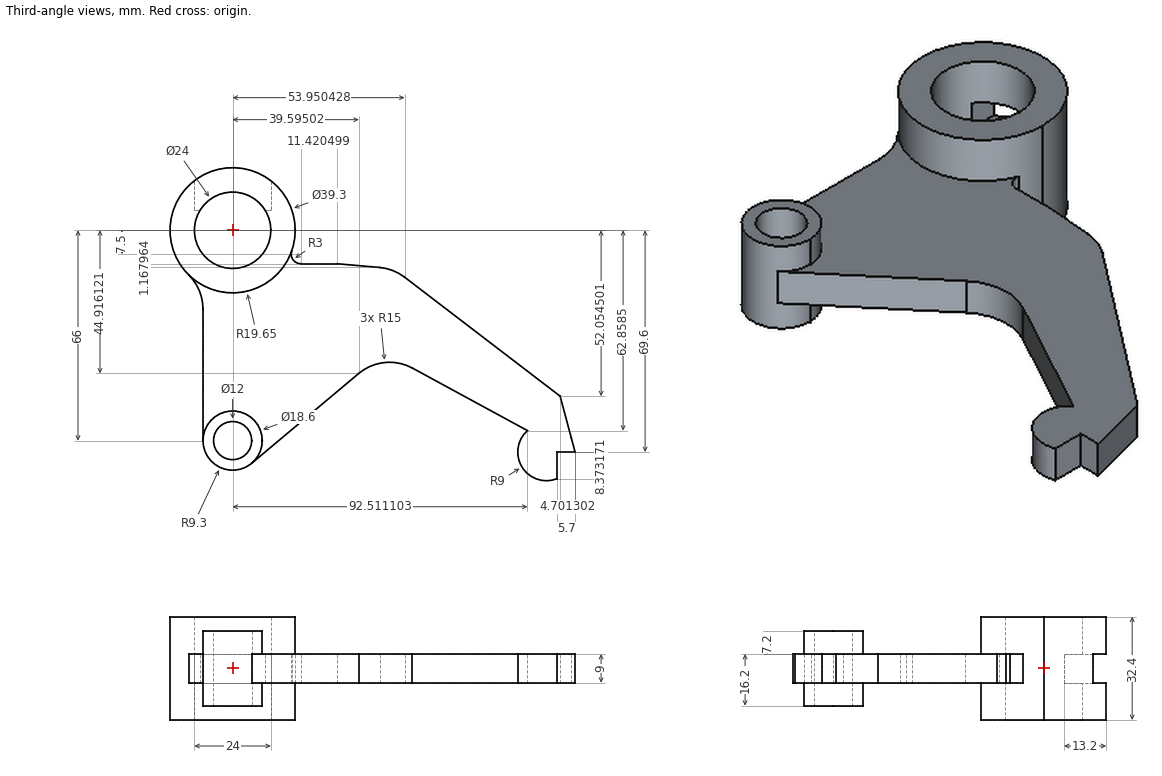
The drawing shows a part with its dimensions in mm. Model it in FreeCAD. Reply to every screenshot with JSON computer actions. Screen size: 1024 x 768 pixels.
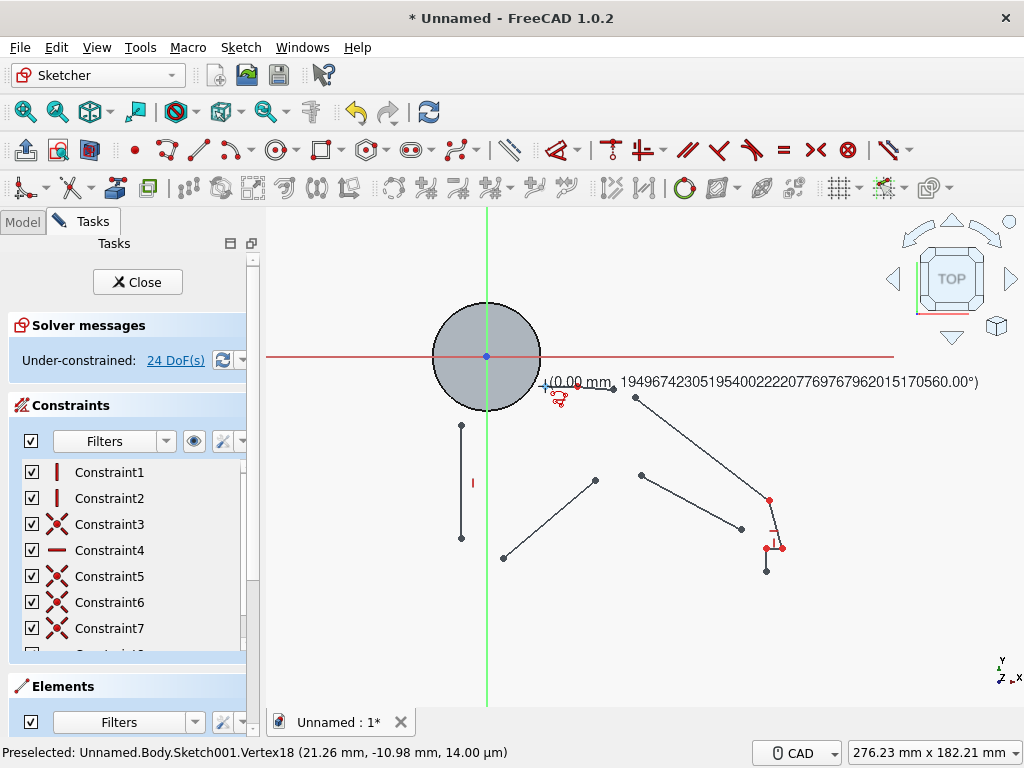
{"action": "key", "text": "g 3 a"}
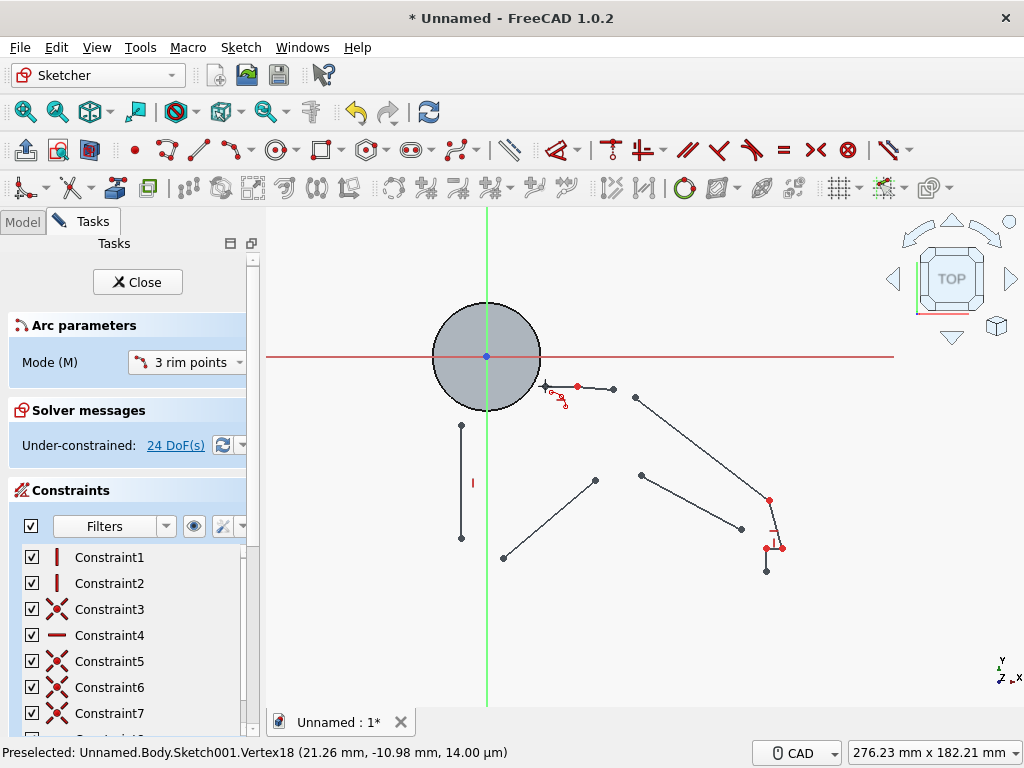
{"action": "left_click", "coordinate": [461, 539]}
{"action": "left_click", "coordinate": [503, 559]}
{"action": "left_click", "coordinate": [471, 558]}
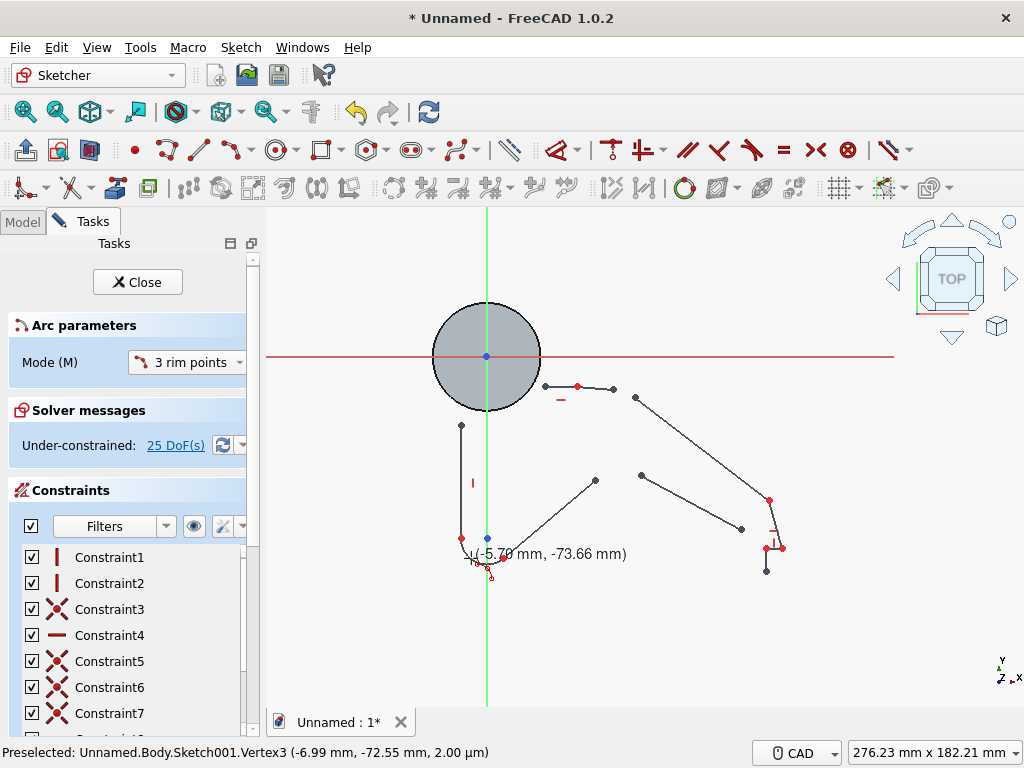
{"action": "left_click", "coordinate": [595, 481]}
{"action": "left_click", "coordinate": [641, 476]}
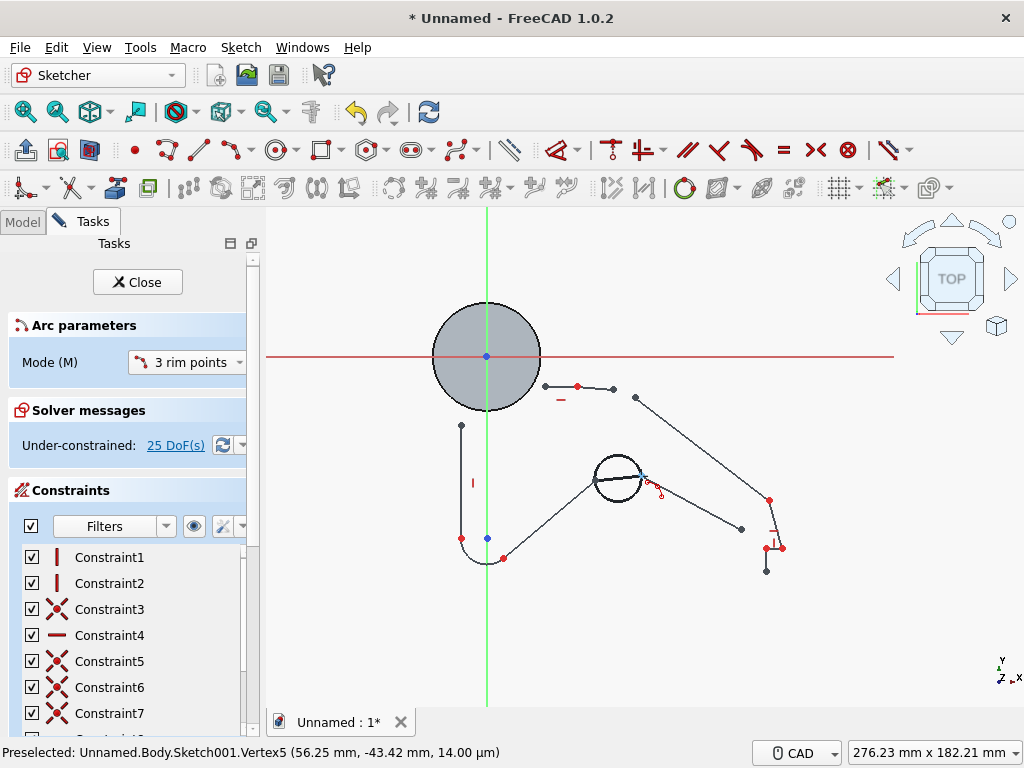
{"action": "scroll", "coordinate": [618, 471], "scroll_direction": "up", "scroll_amount": 4}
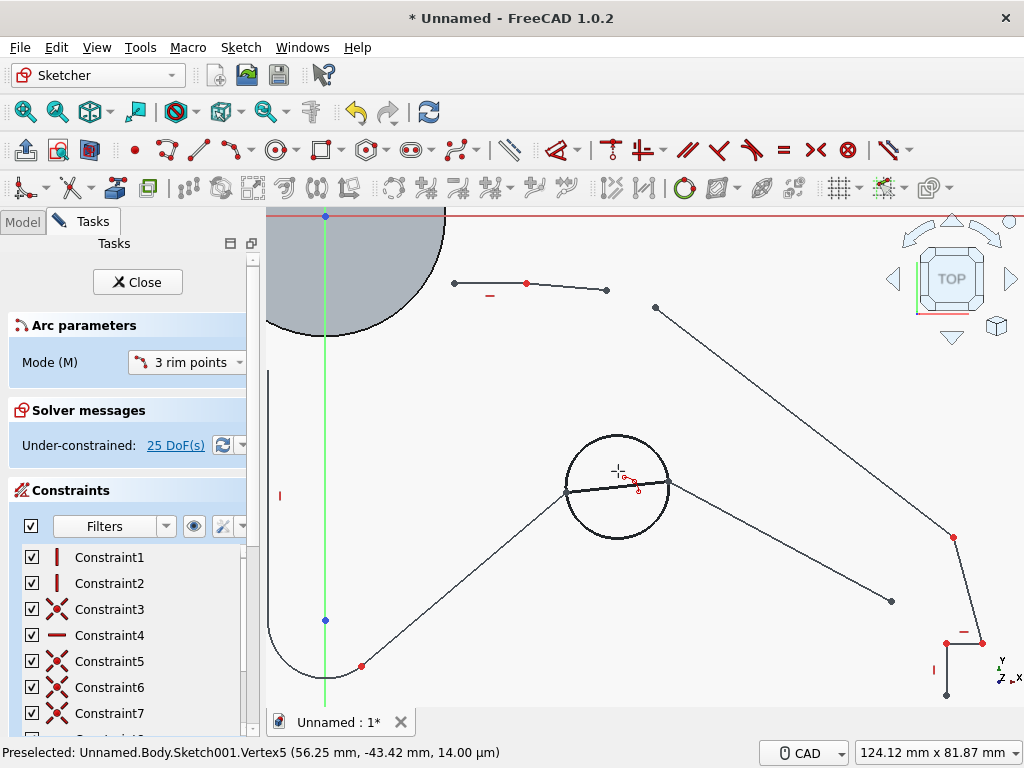
{"action": "left_click", "coordinate": [617, 470]}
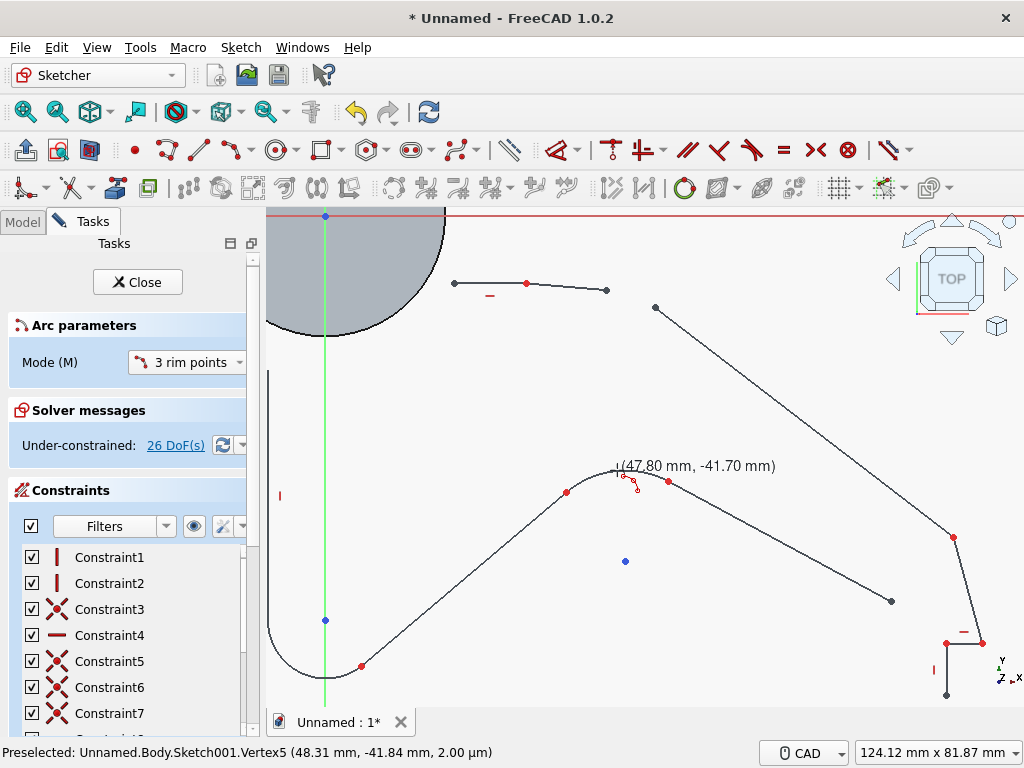
{"action": "scroll", "coordinate": [534, 460], "scroll_direction": "down", "scroll_amount": 3}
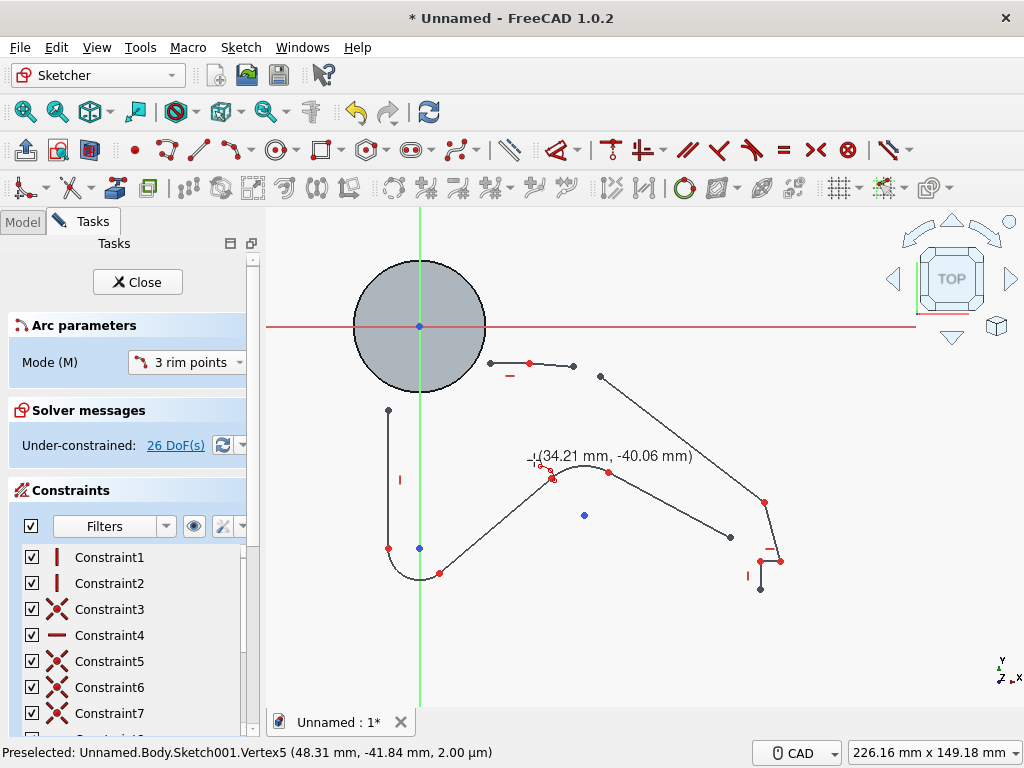
{"action": "left_click", "coordinate": [730, 538]}
{"action": "left_click", "coordinate": [761, 589]}
{"action": "left_click", "coordinate": [724, 576]}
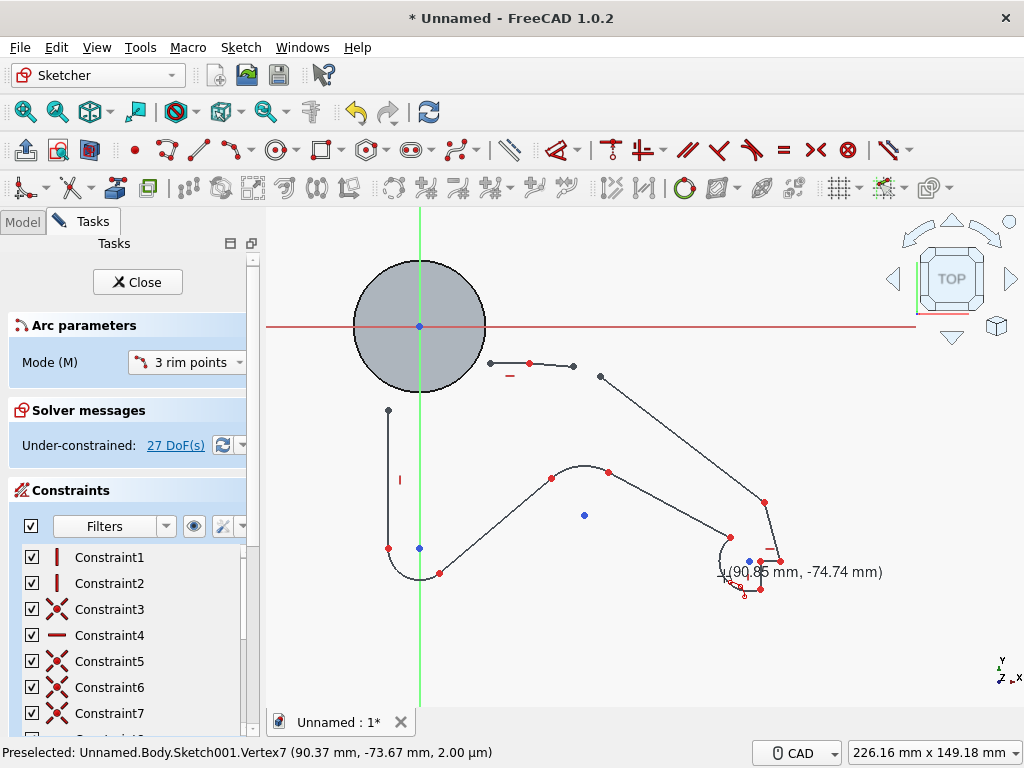
{"action": "left_click", "coordinate": [601, 377]}
{"action": "left_click", "coordinate": [574, 367]}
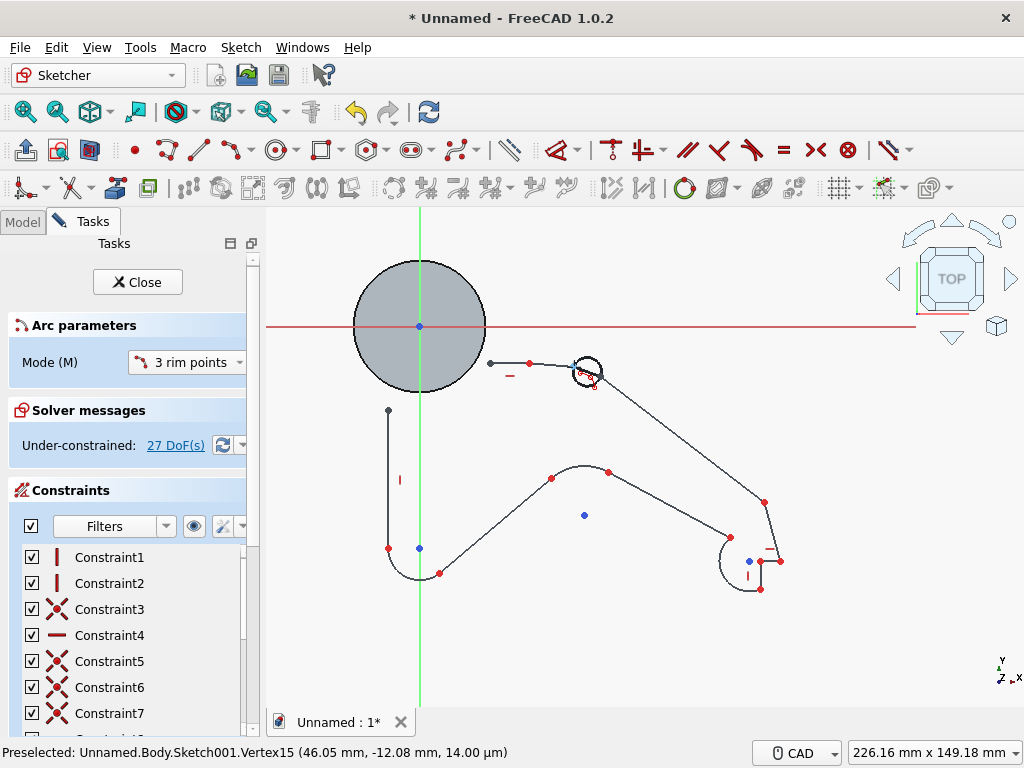
{"action": "scroll", "coordinate": [588, 369], "scroll_direction": "up", "scroll_amount": 11}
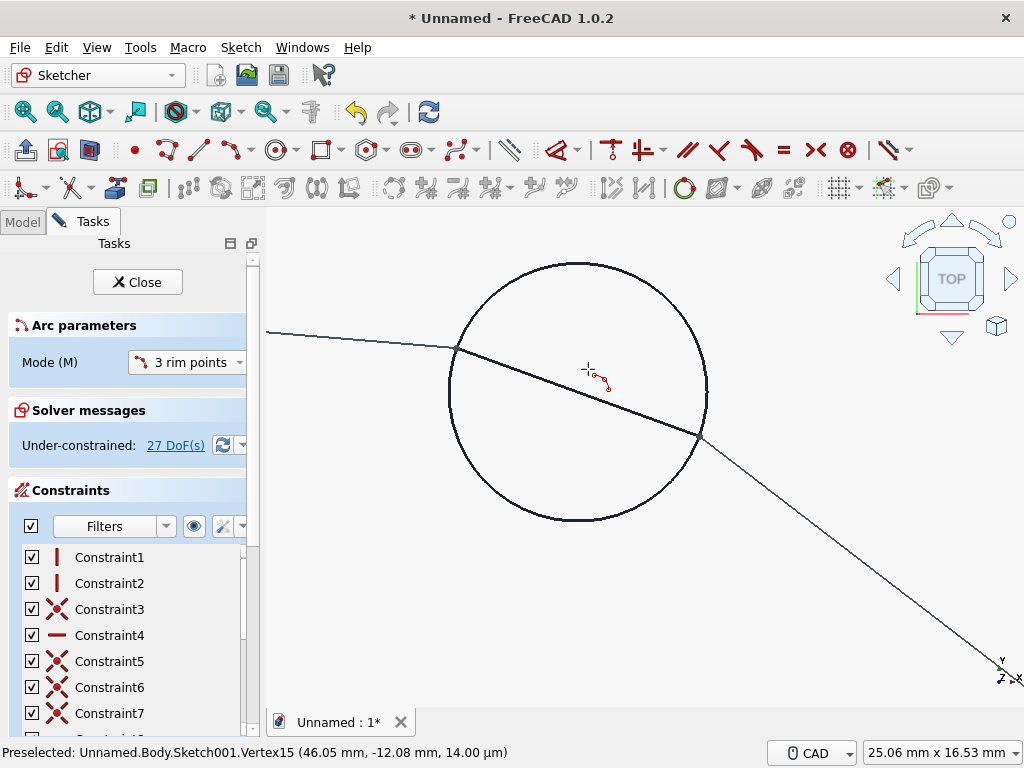
{"action": "left_click", "coordinate": [584, 365]}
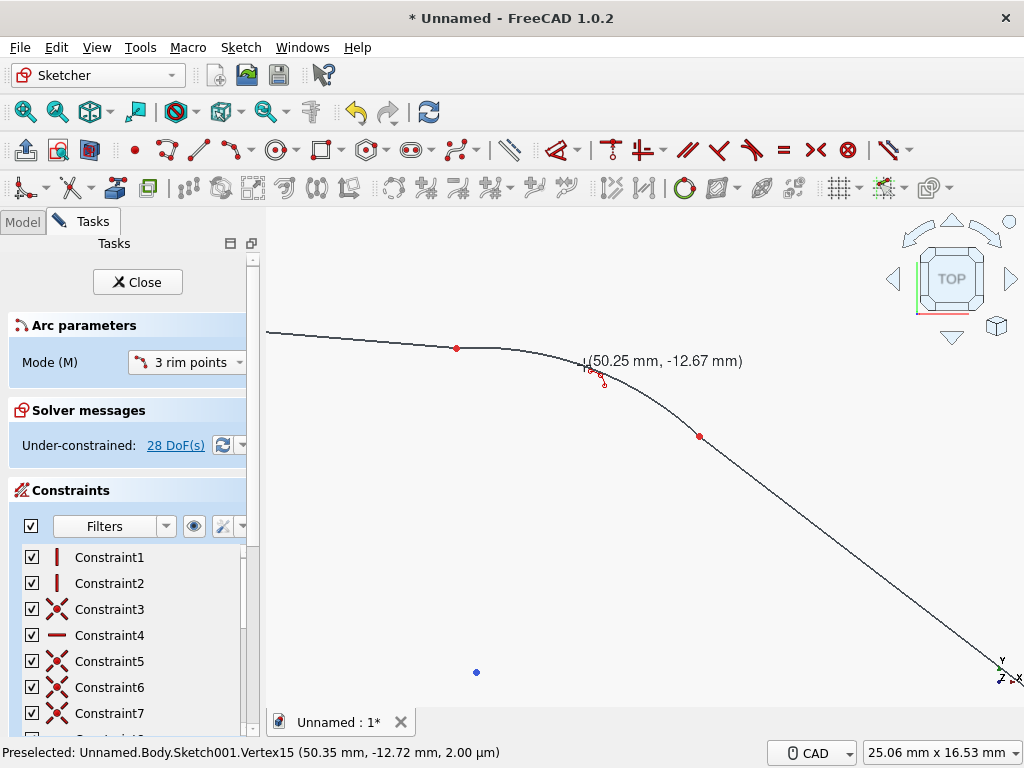
{"action": "scroll", "coordinate": [588, 369], "scroll_direction": "down", "scroll_amount": 11}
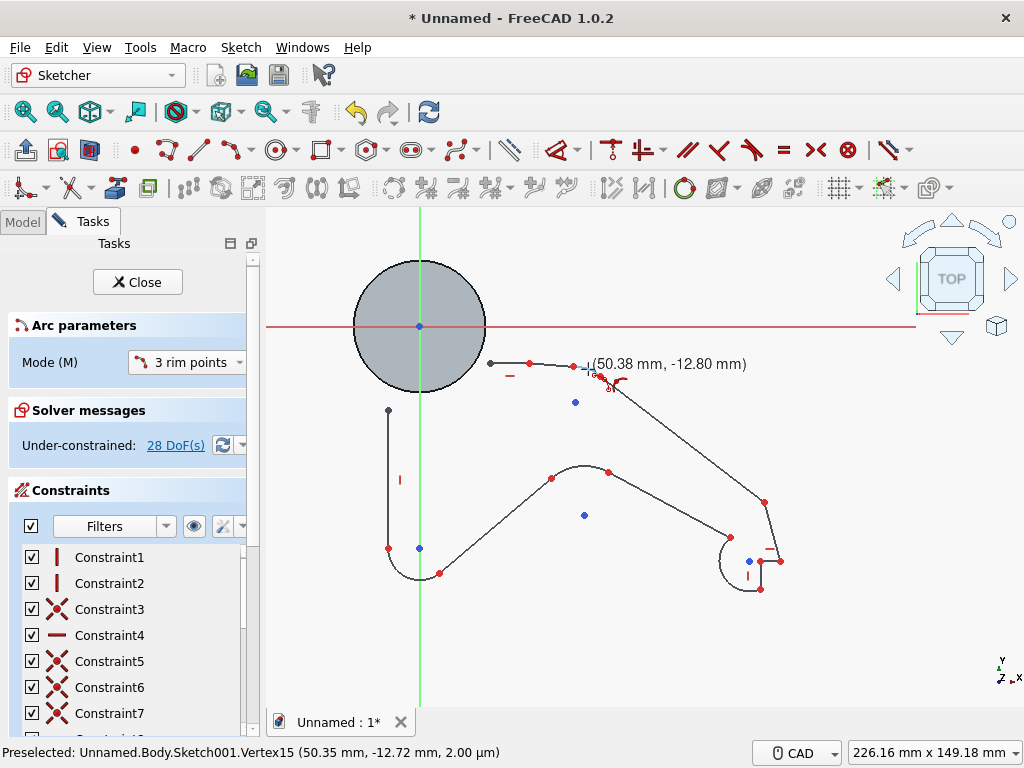
{"action": "left_click", "coordinate": [491, 363]}
{"action": "left_click", "coordinate": [482, 348]}